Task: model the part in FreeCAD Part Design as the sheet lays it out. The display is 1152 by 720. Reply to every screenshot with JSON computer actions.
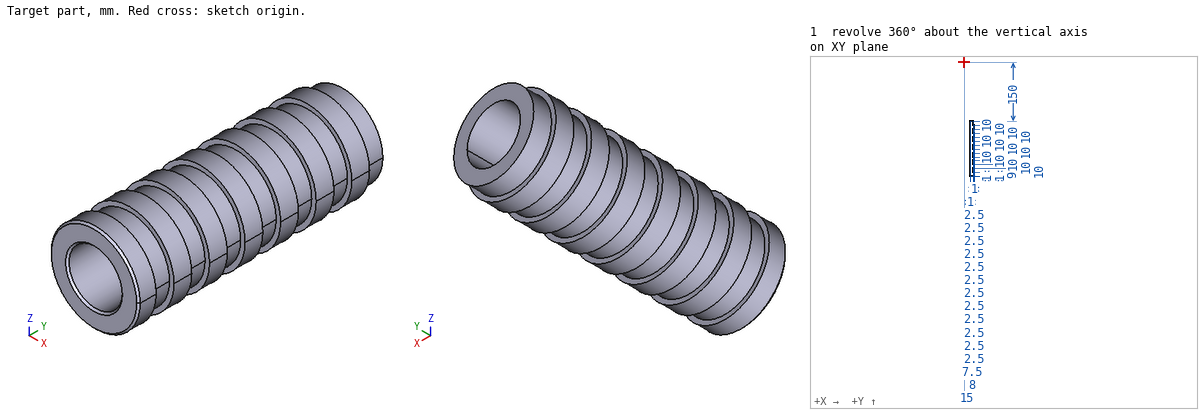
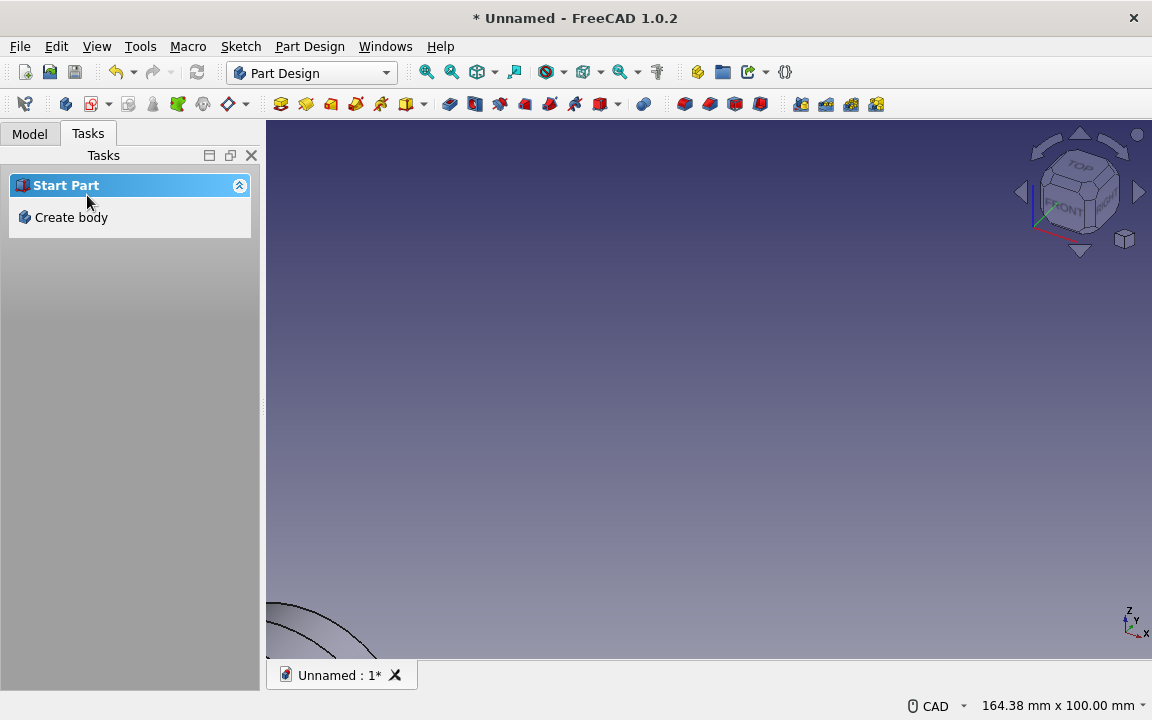
{"action": "key", "text": "0"}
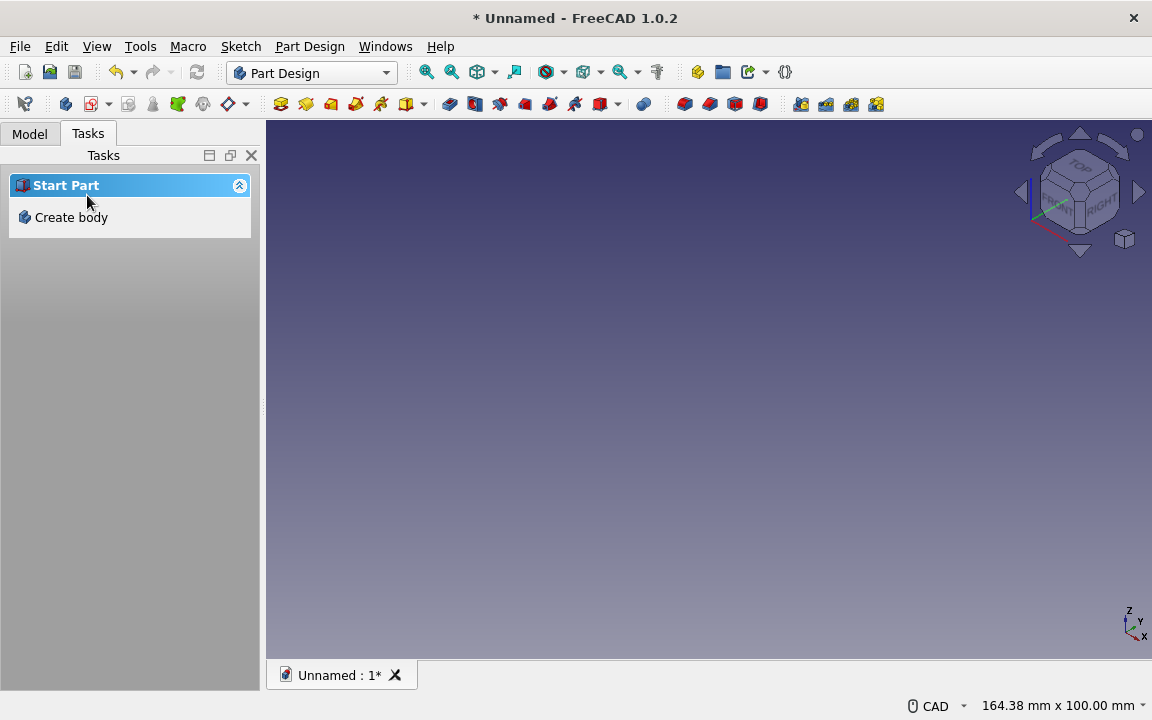
{"action": "left_click", "coordinate": [427, 72]}